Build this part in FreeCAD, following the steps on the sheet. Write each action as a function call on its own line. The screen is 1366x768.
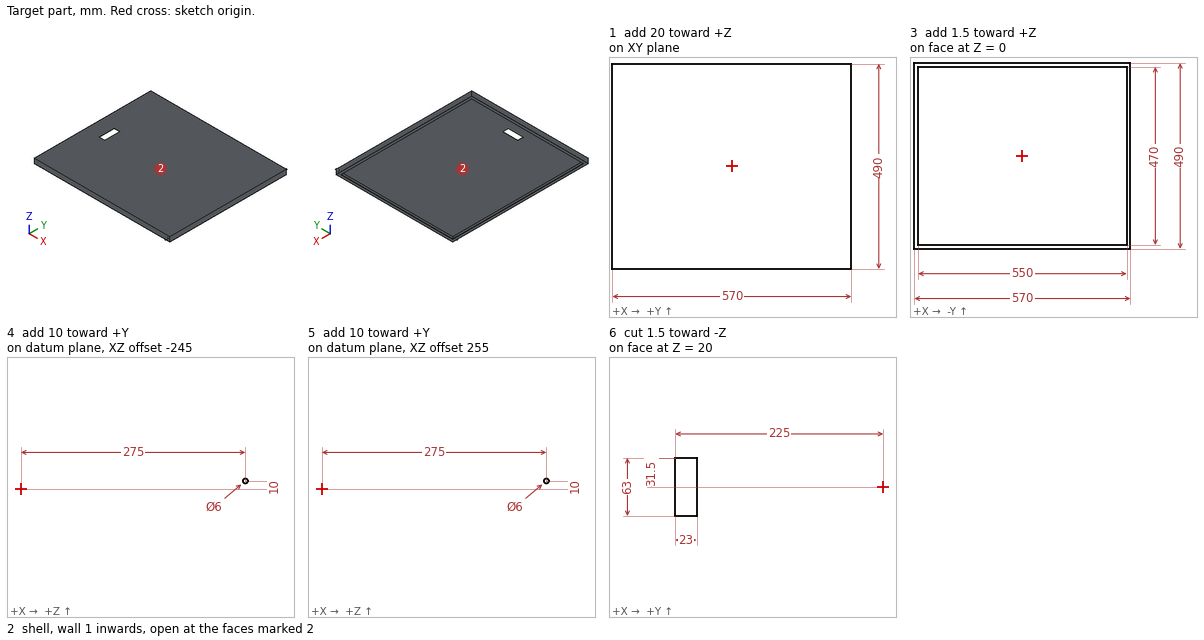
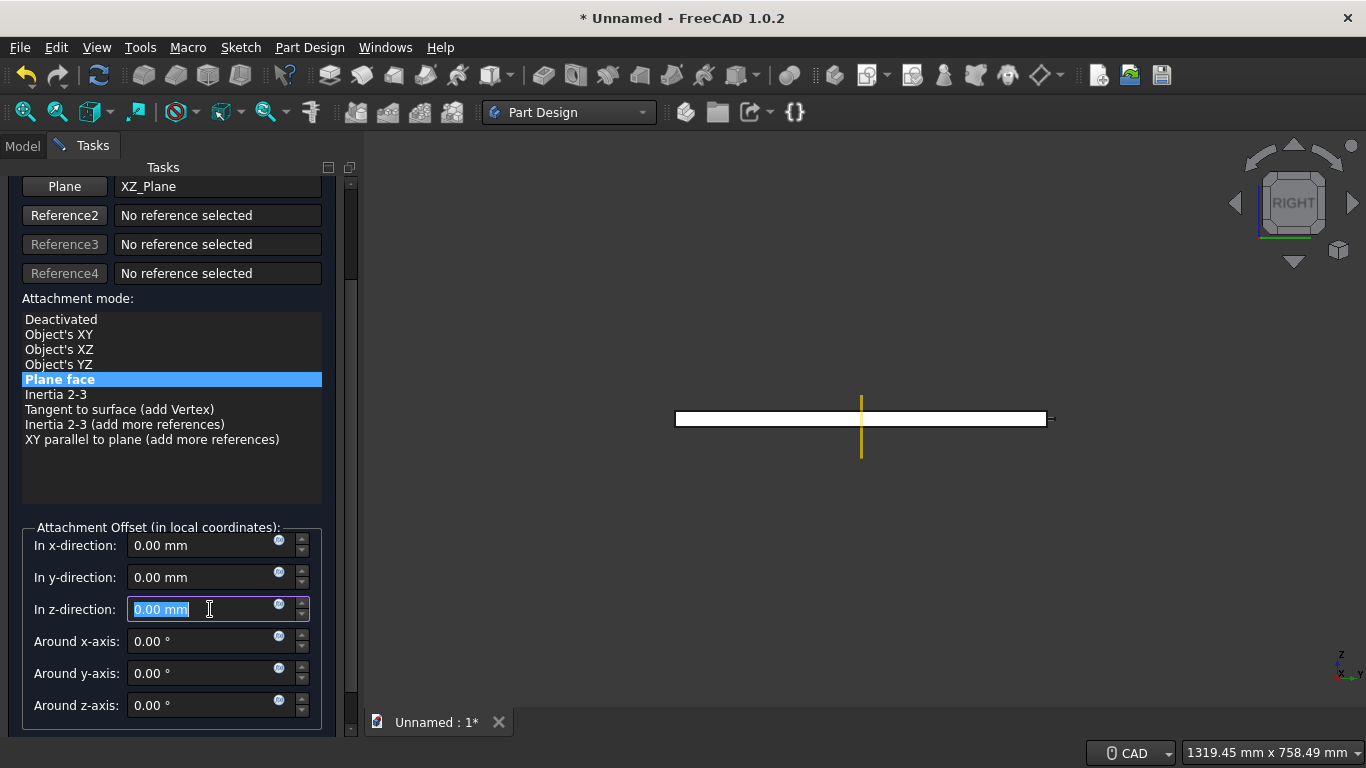
text(255)
key(Tab)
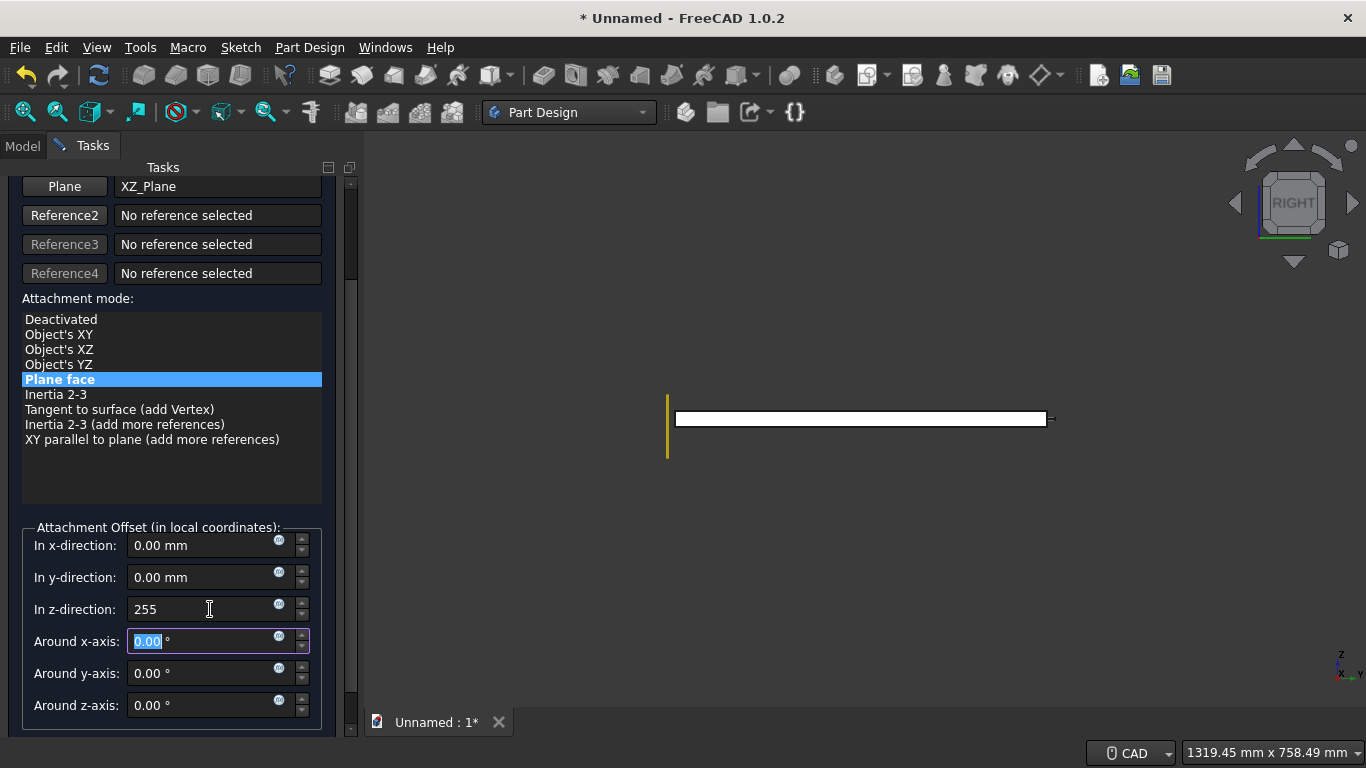
scroll(351, 456, up, 3)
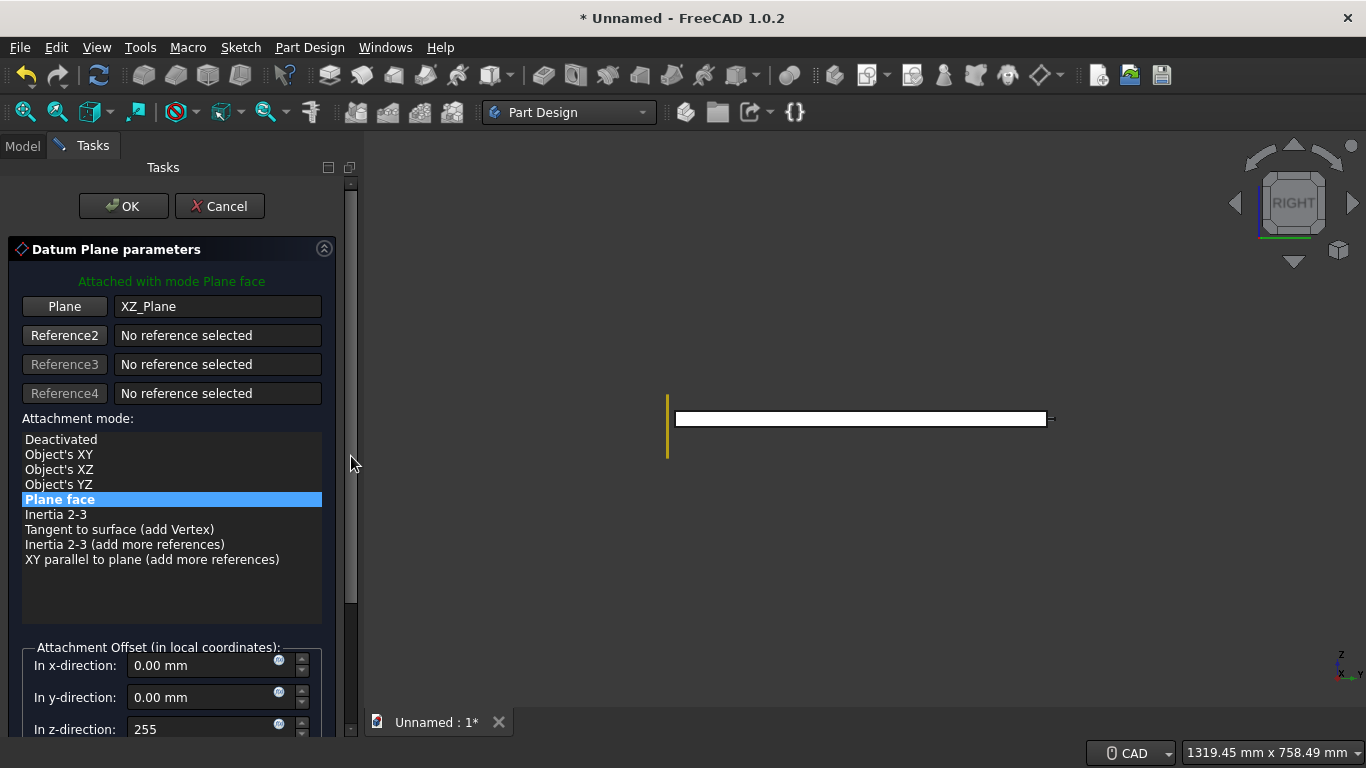
click(124, 206)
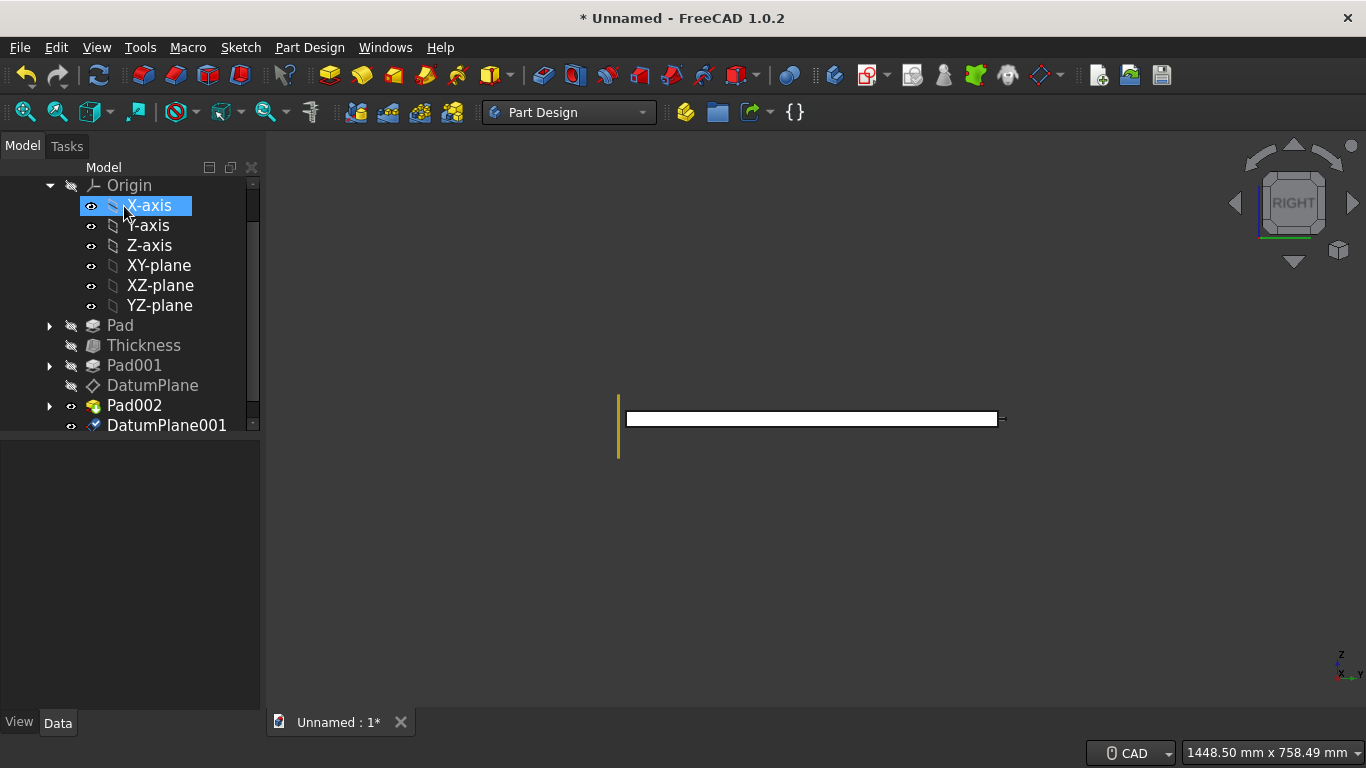
click(116, 426)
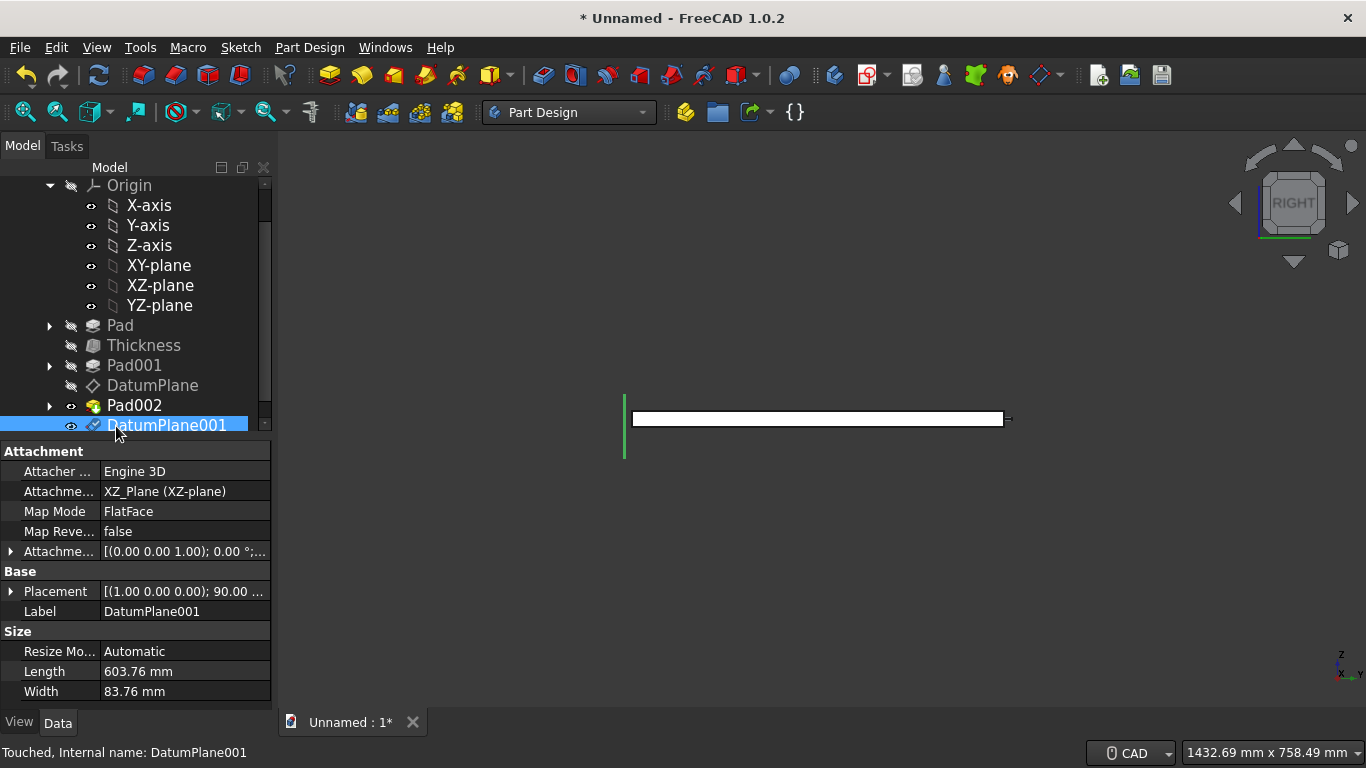
click(868, 76)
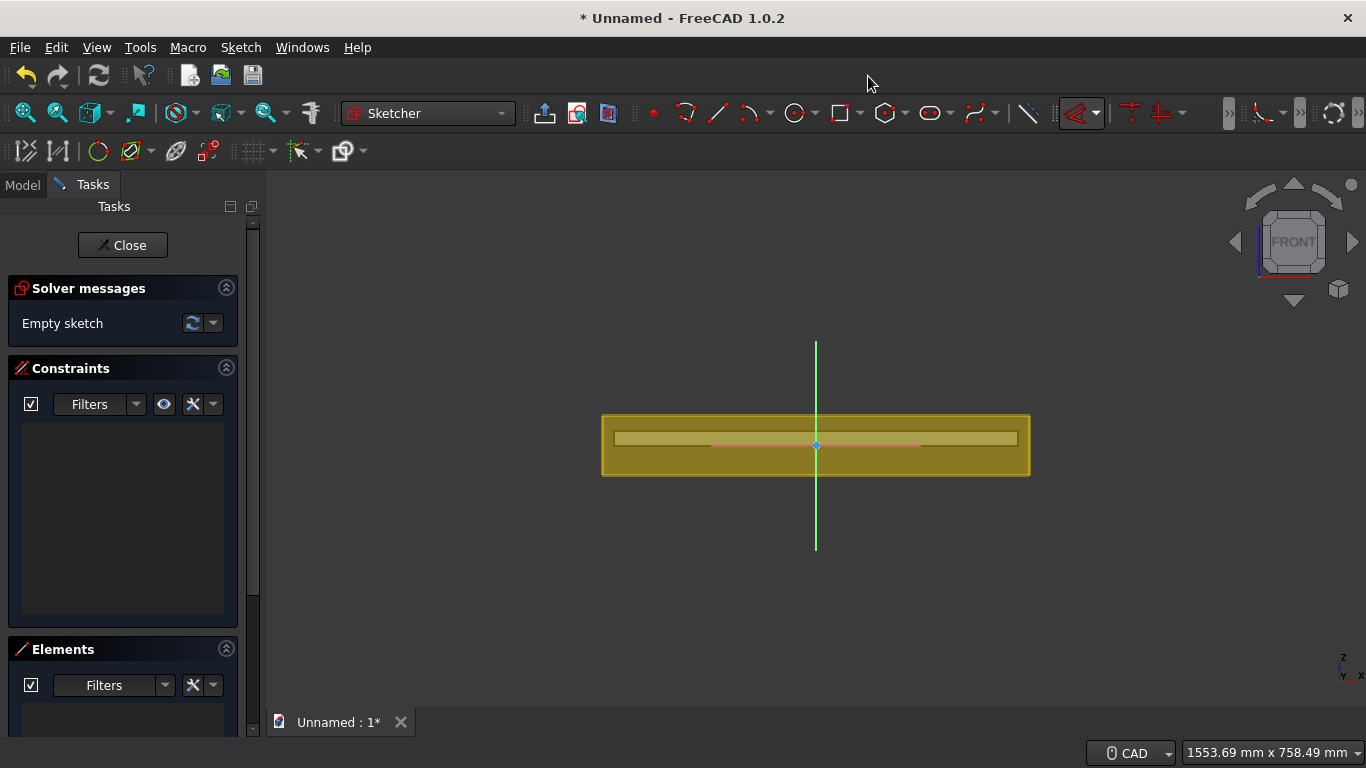
scroll(1024, 438, up, 15)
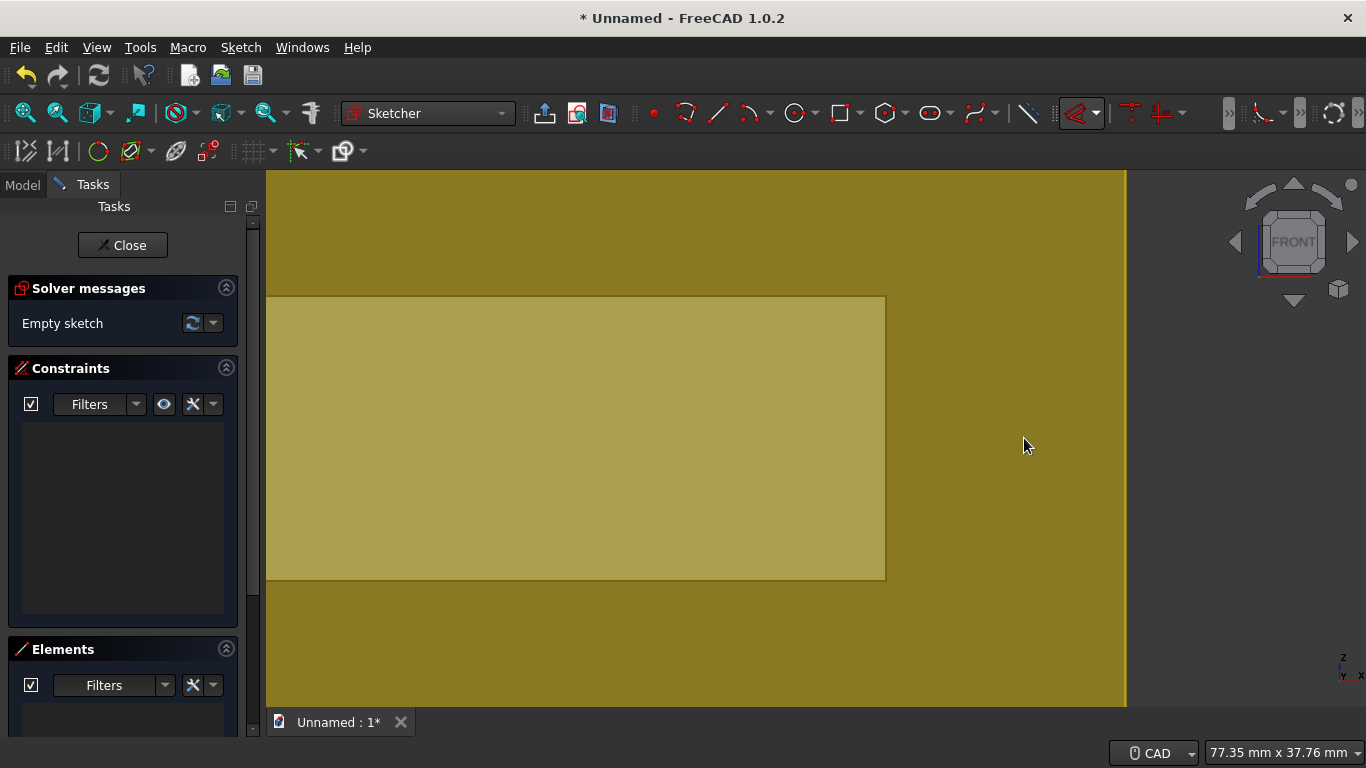
scroll(742, 438, up, 7)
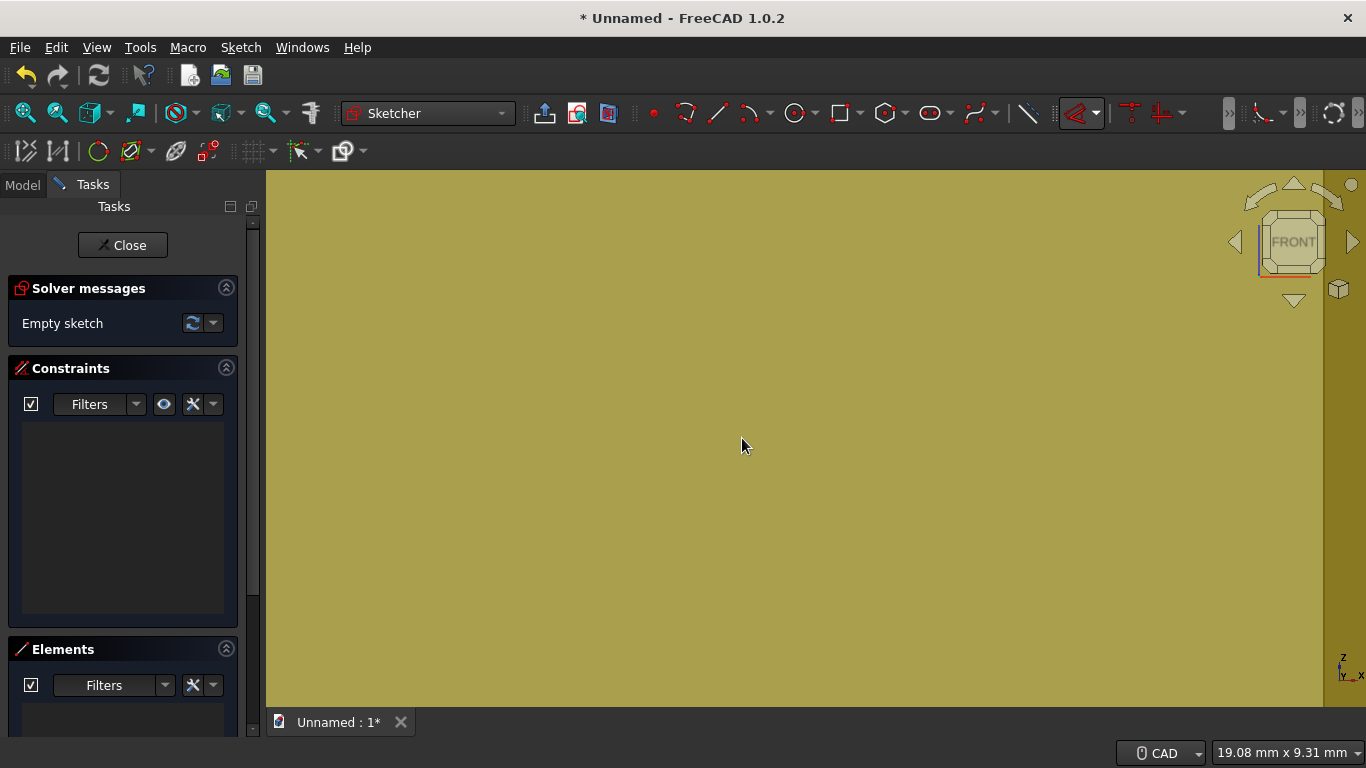
key(g)
key(c)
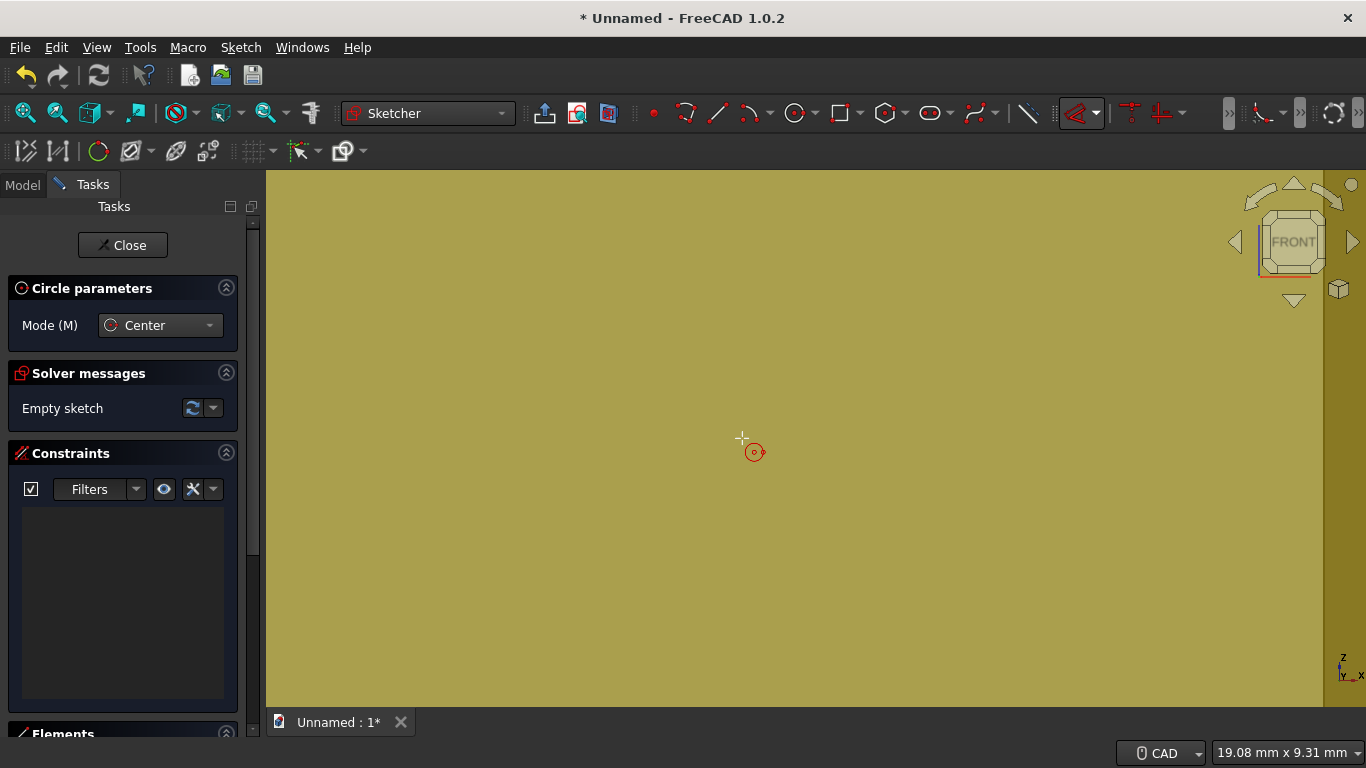
click(747, 438)
click(870, 316)
key(Escape)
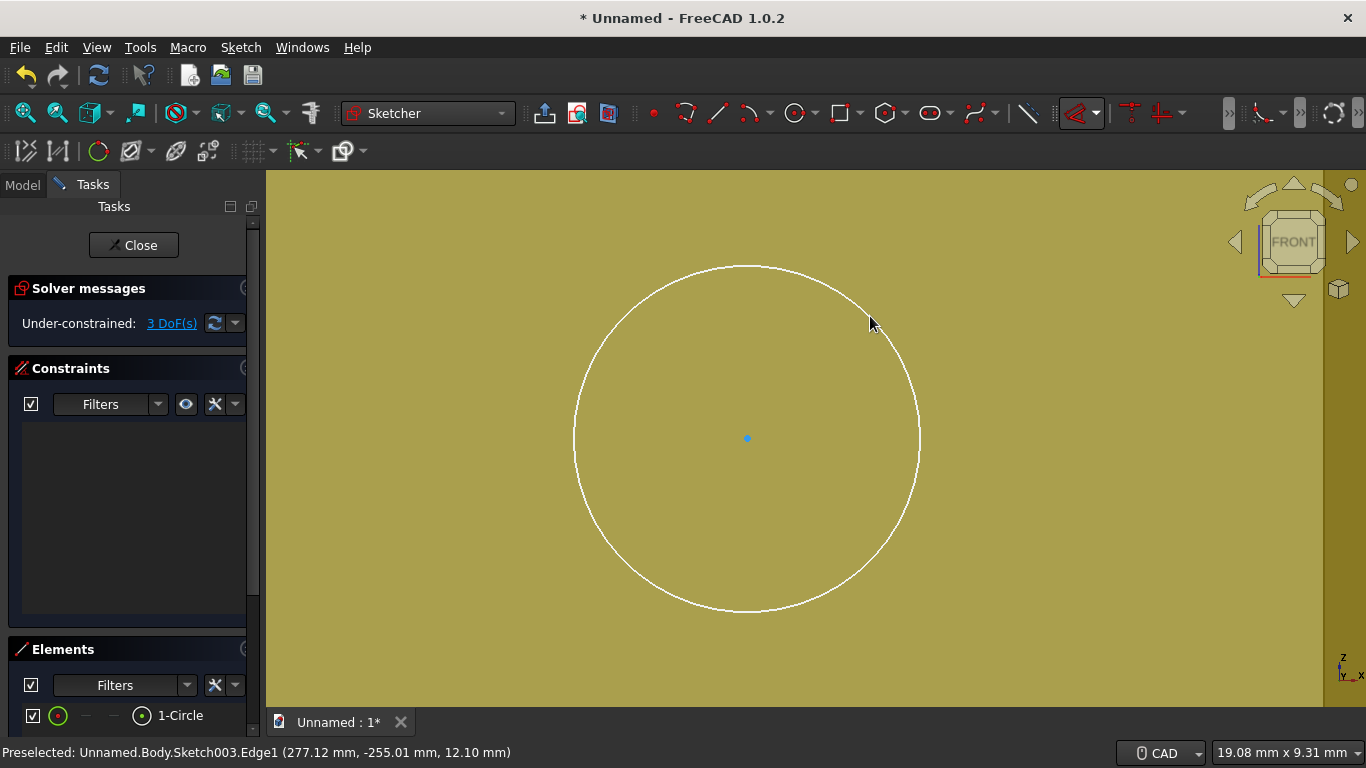
click(869, 316)